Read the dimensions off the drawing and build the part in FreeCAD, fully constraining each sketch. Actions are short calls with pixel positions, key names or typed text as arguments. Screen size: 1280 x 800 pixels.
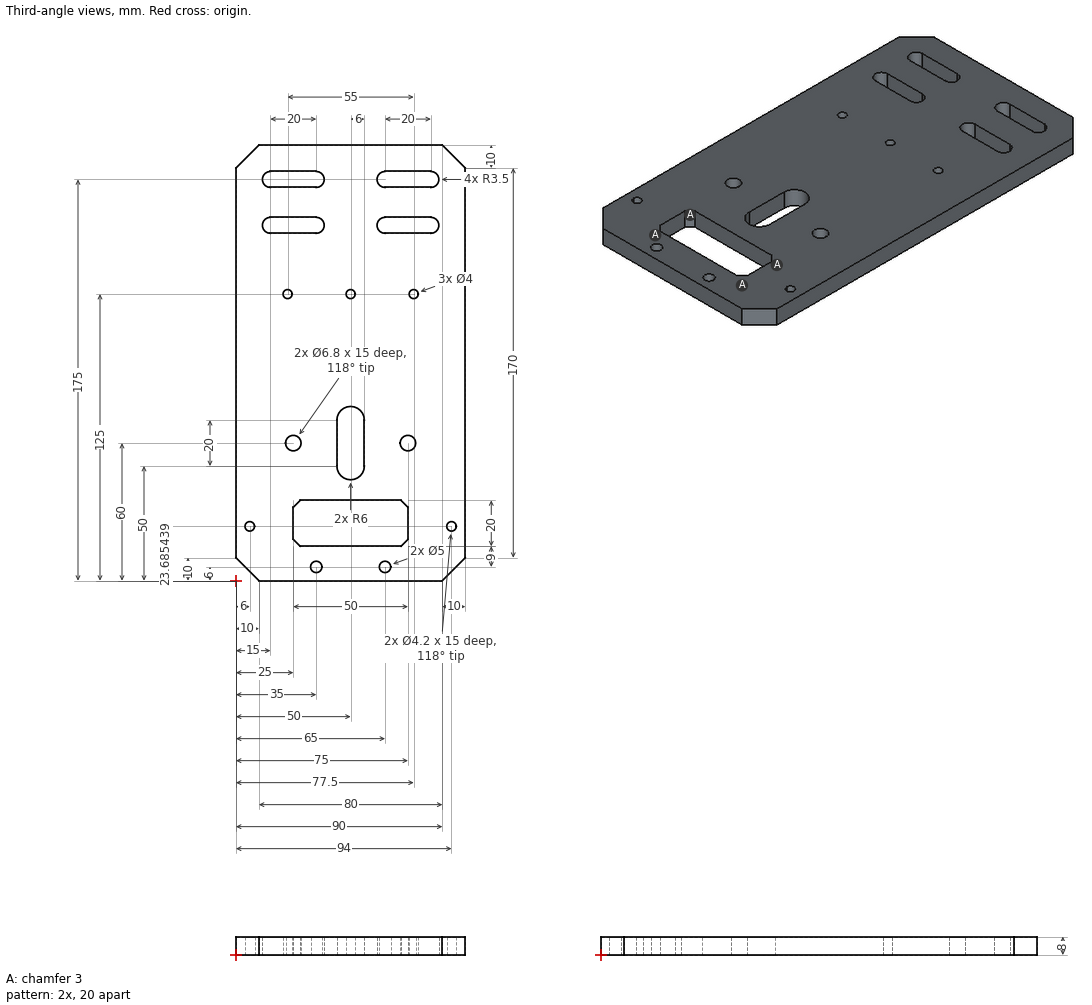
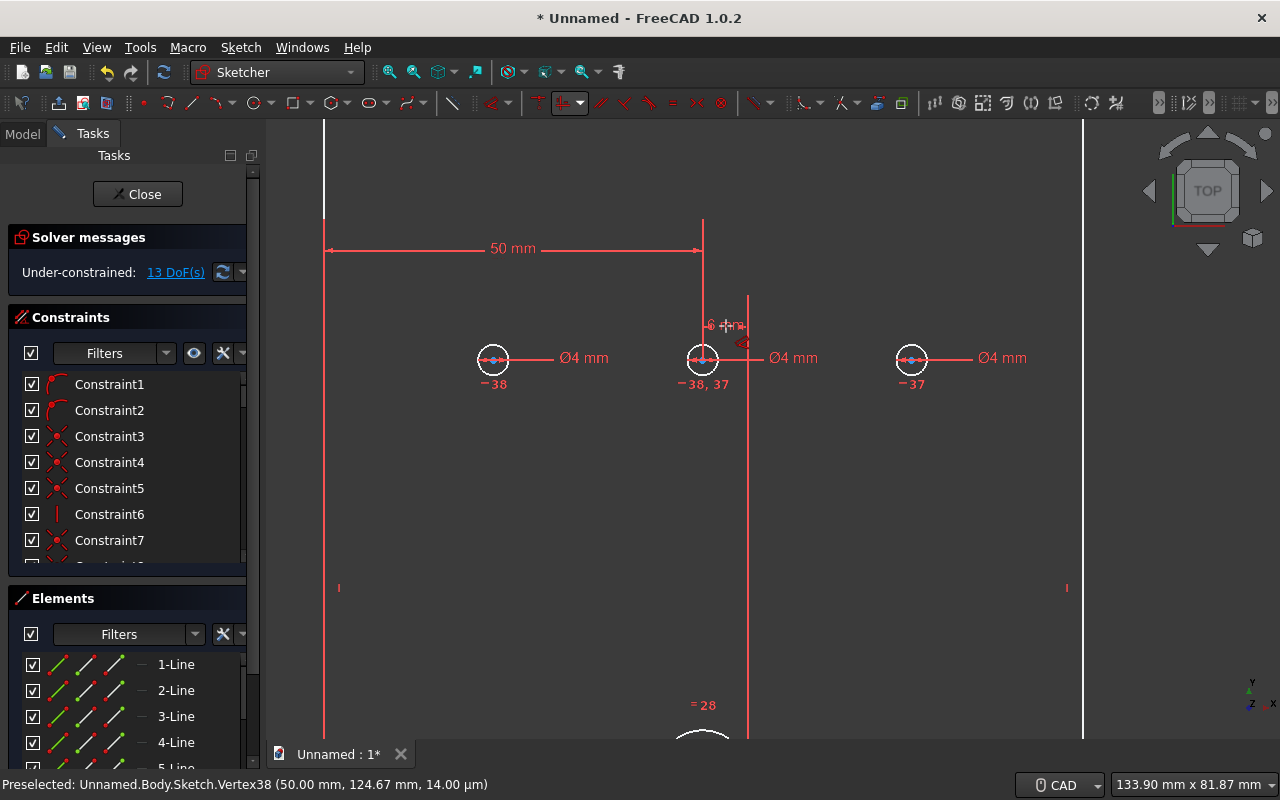
click(1083, 330)
click(1049, 429)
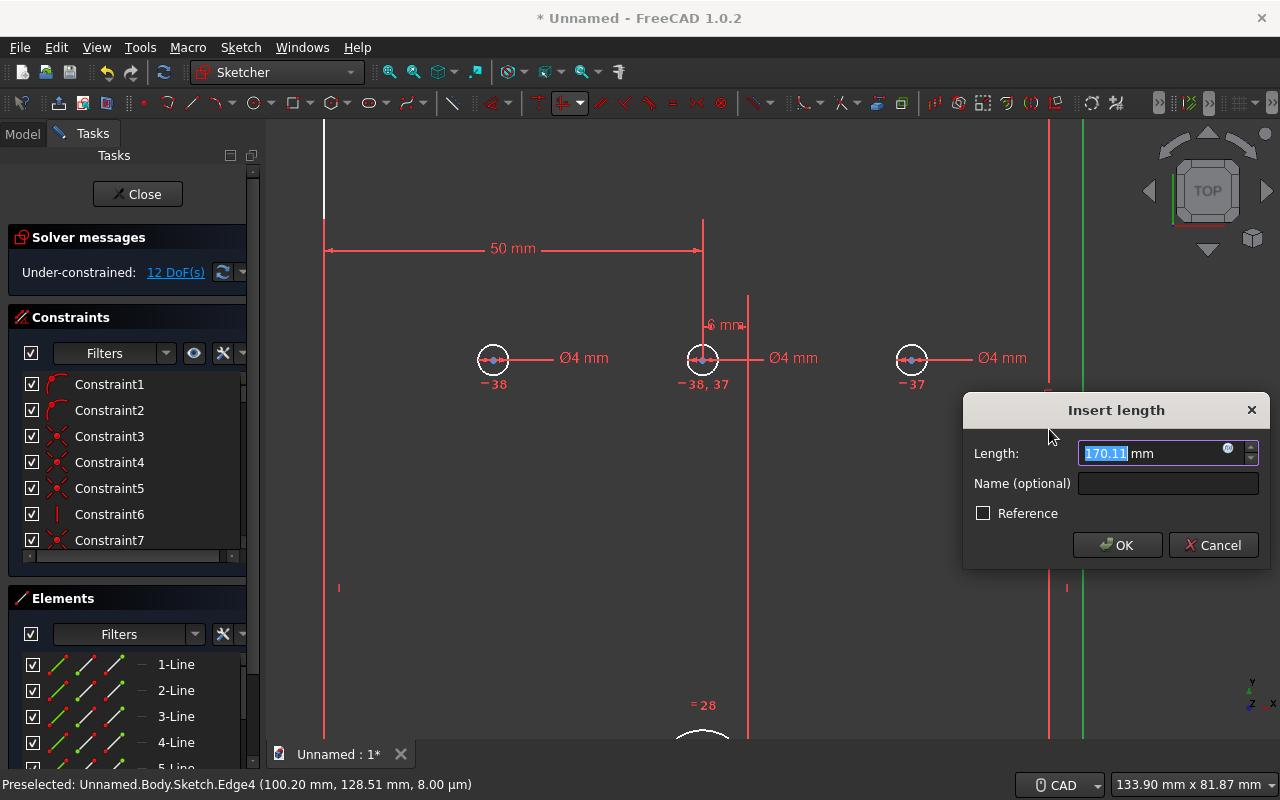
text(170)
key(Return)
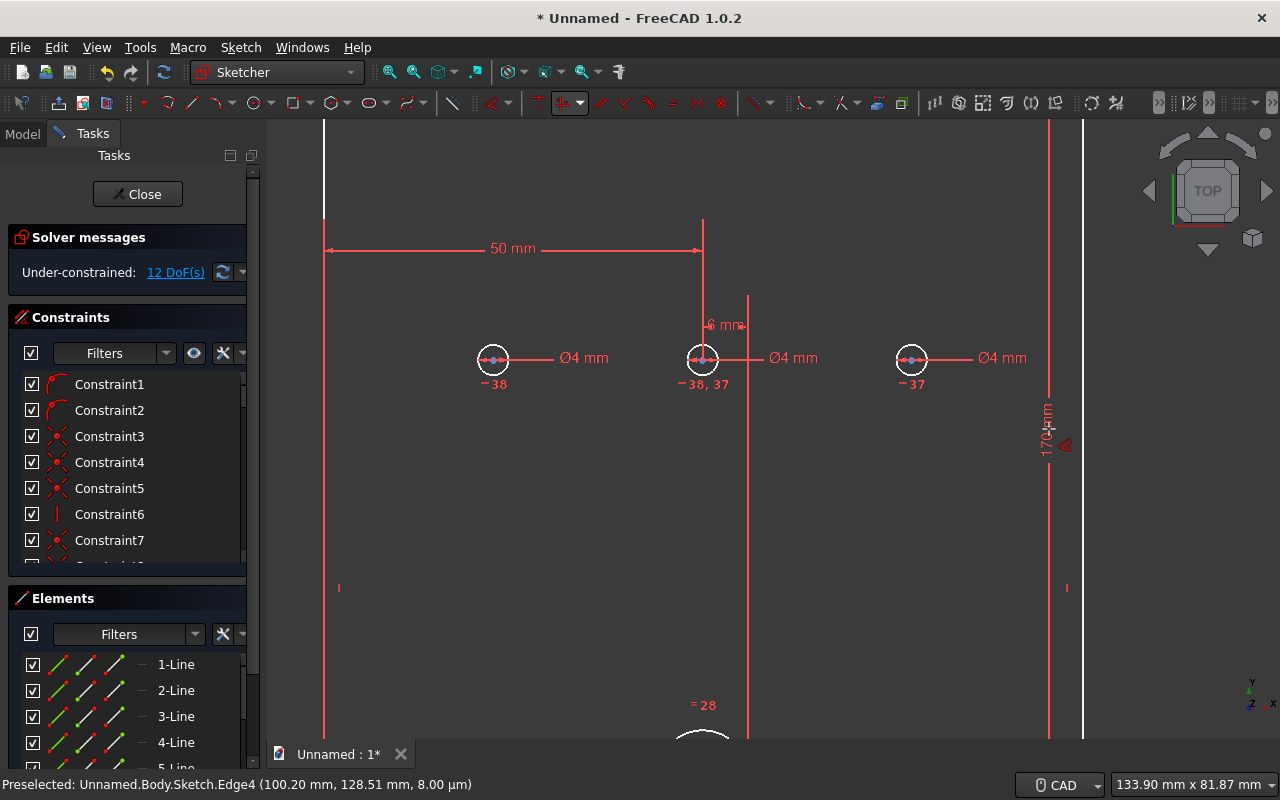
click(324, 330)
click(358, 429)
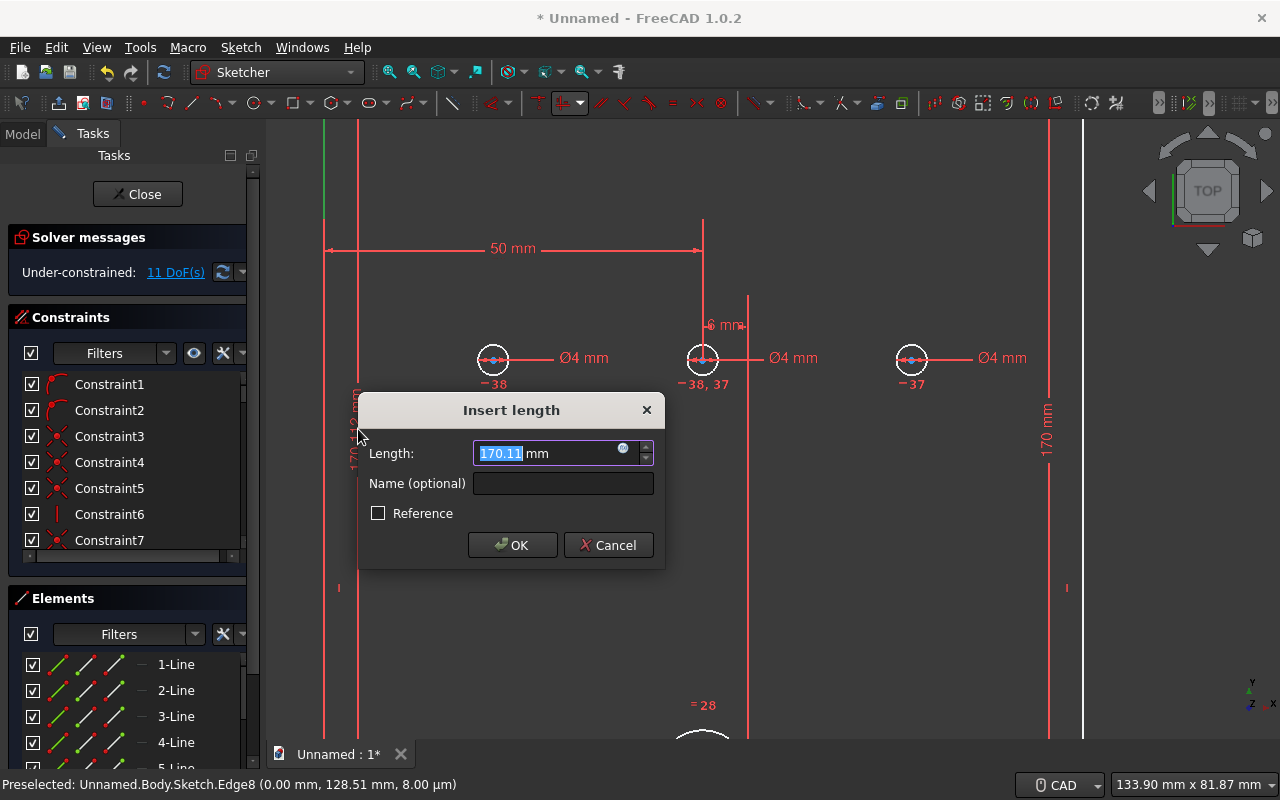
text(170)
key(Return)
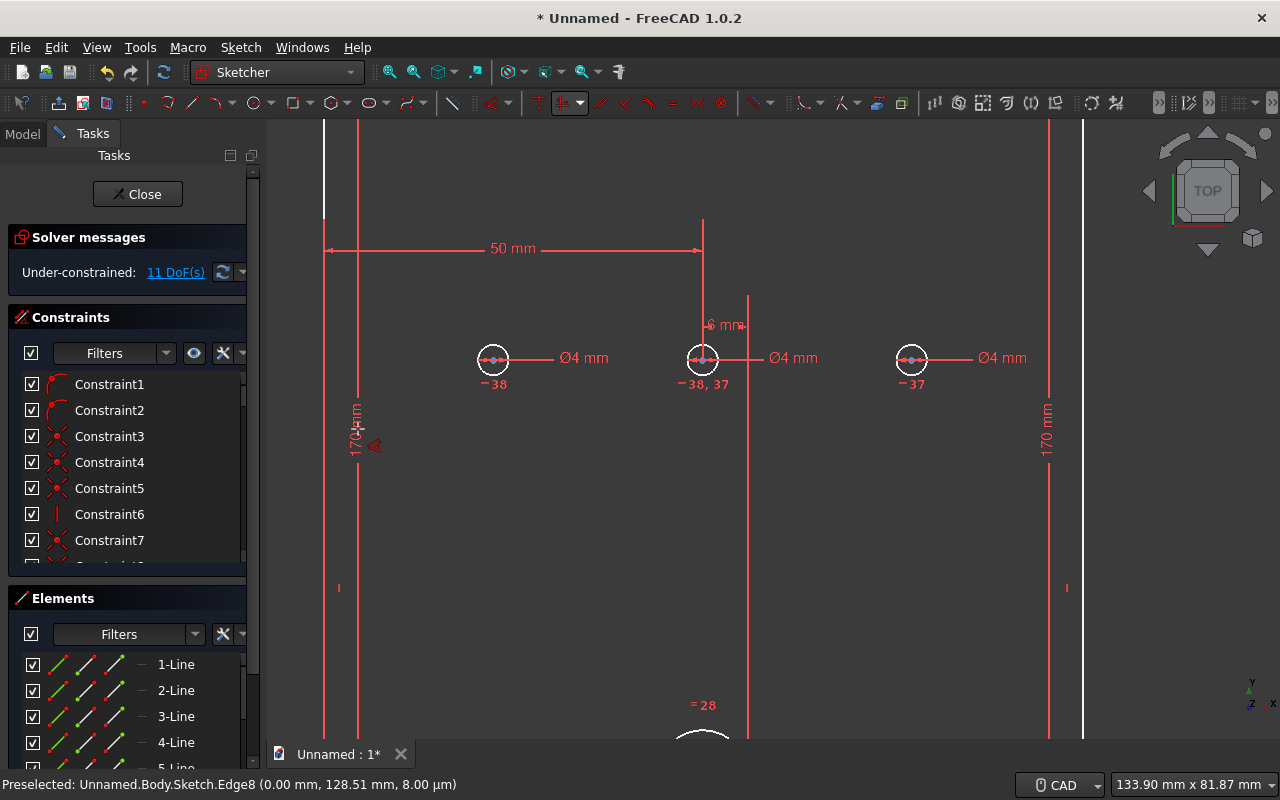
scroll(705, 362, down, 6)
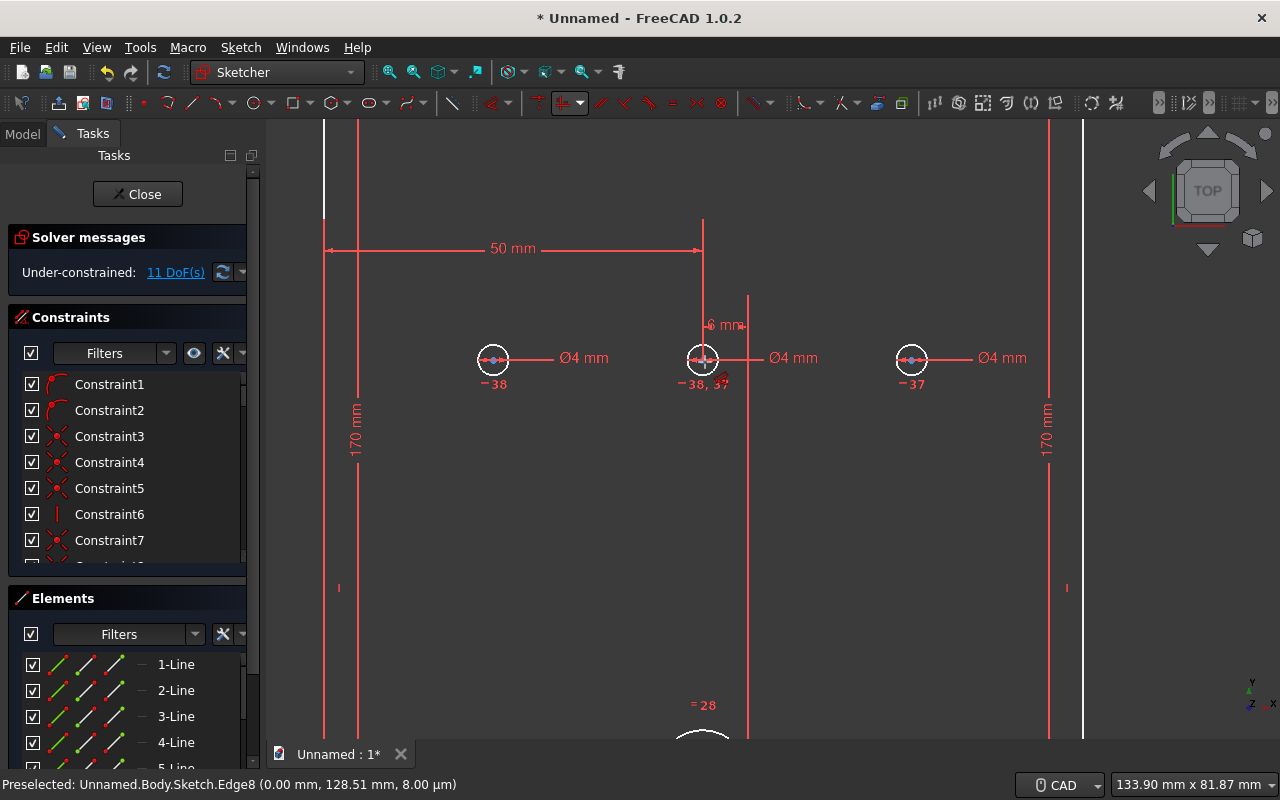
scroll(591, 624, up, 3)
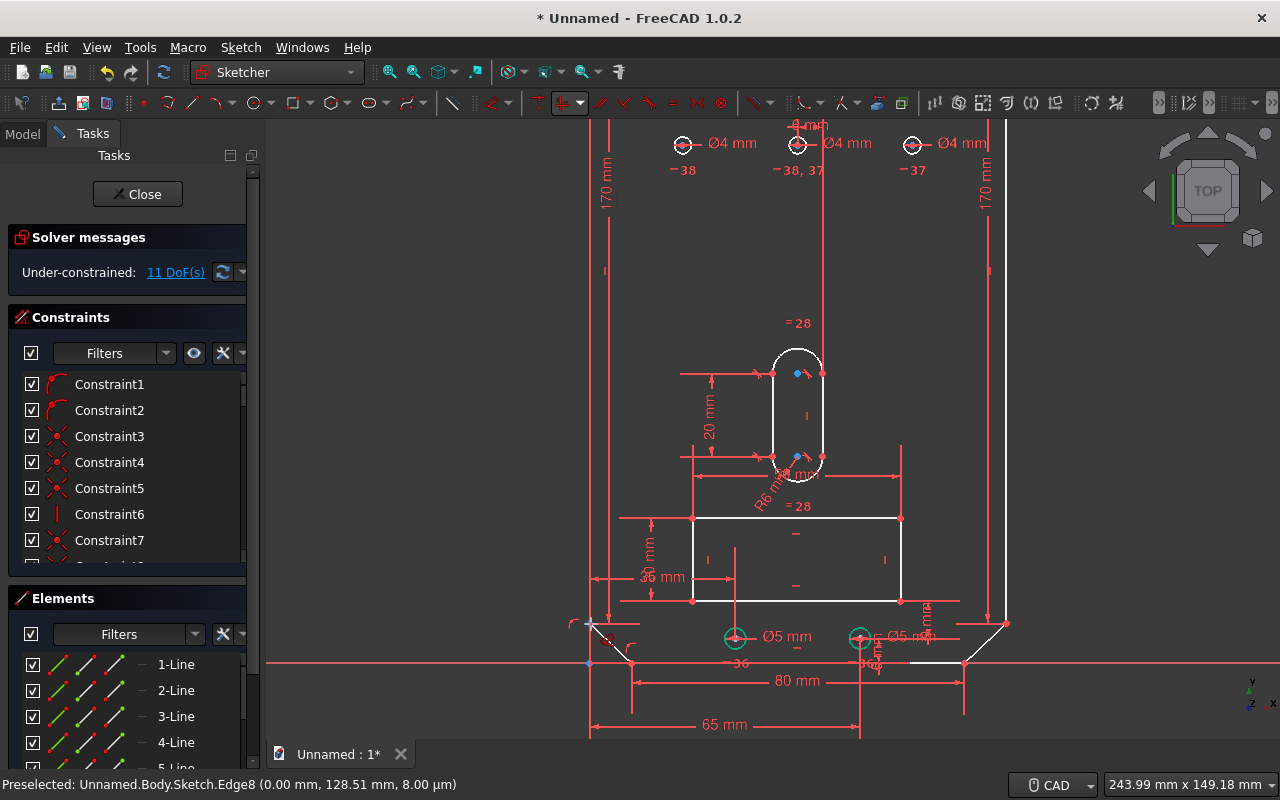
click(590, 624)
click(556, 644)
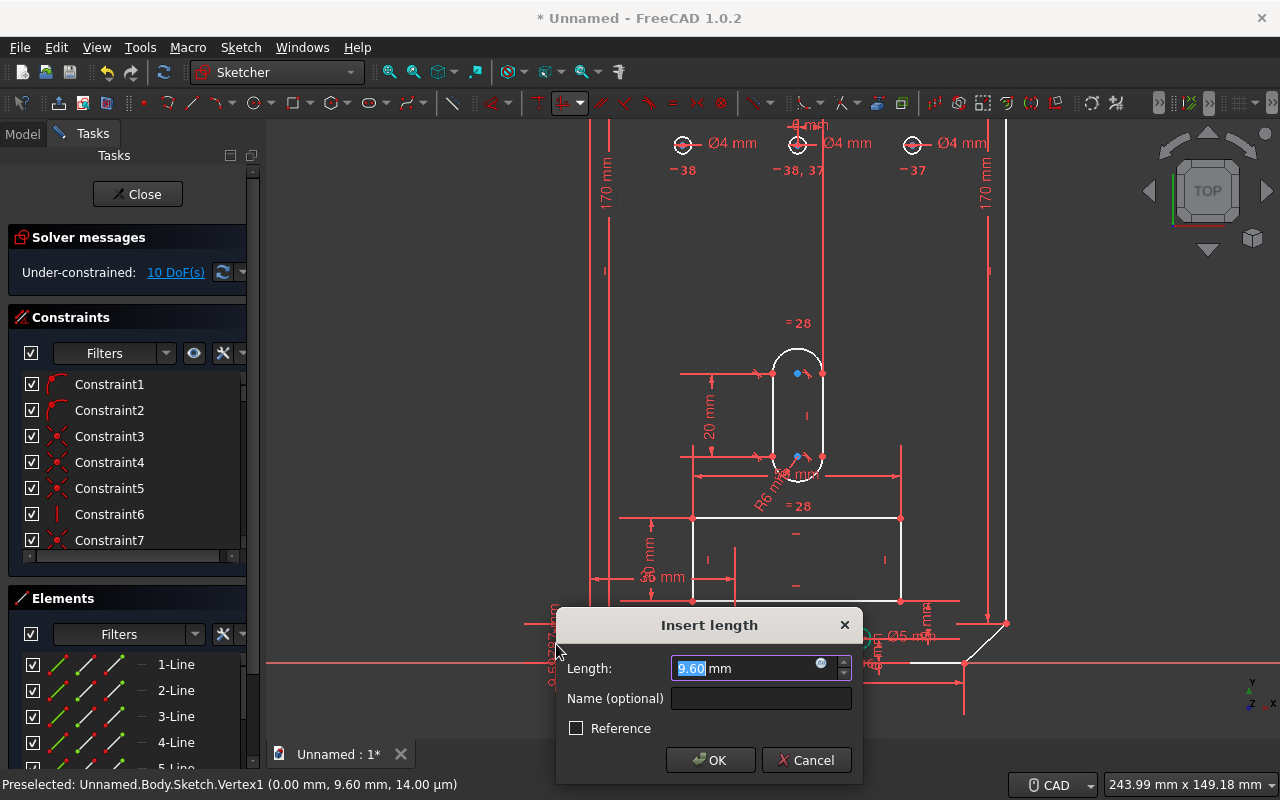
text(10)
key(Return)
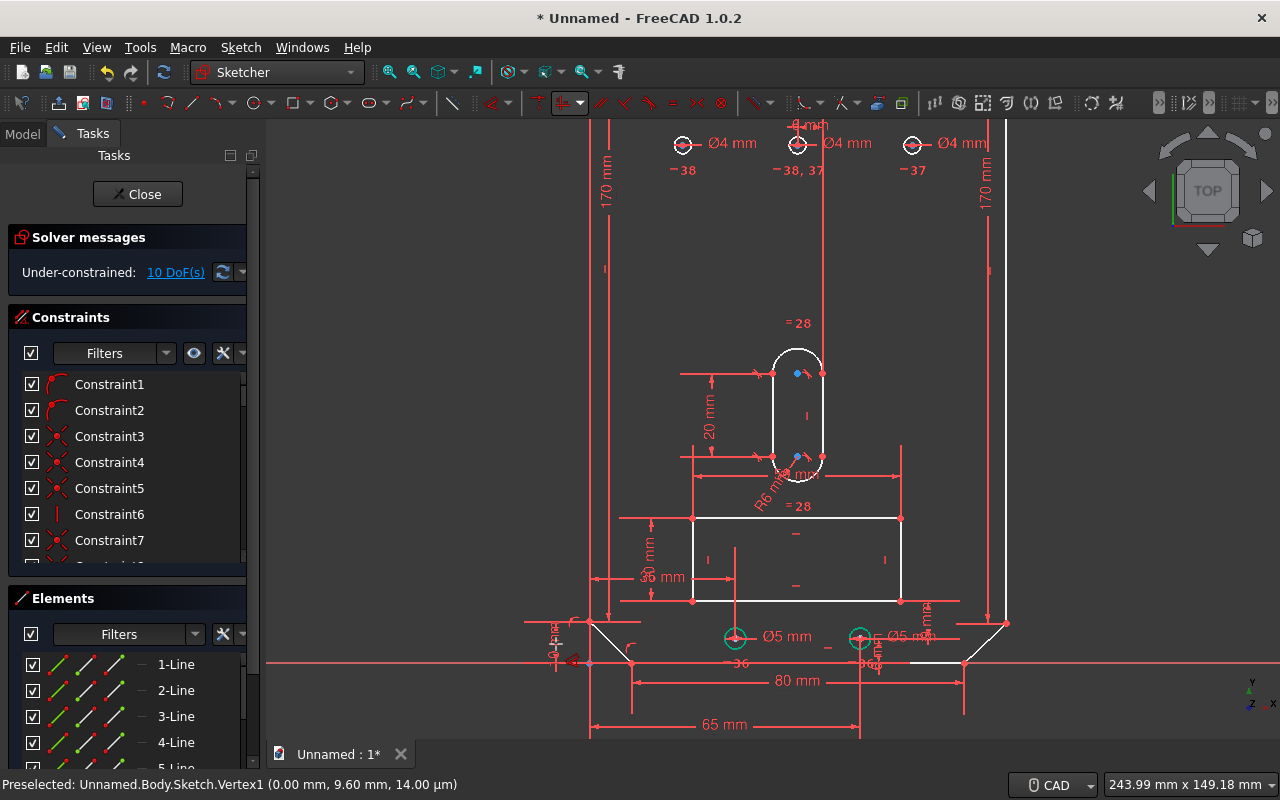
click(632, 663)
click(611, 697)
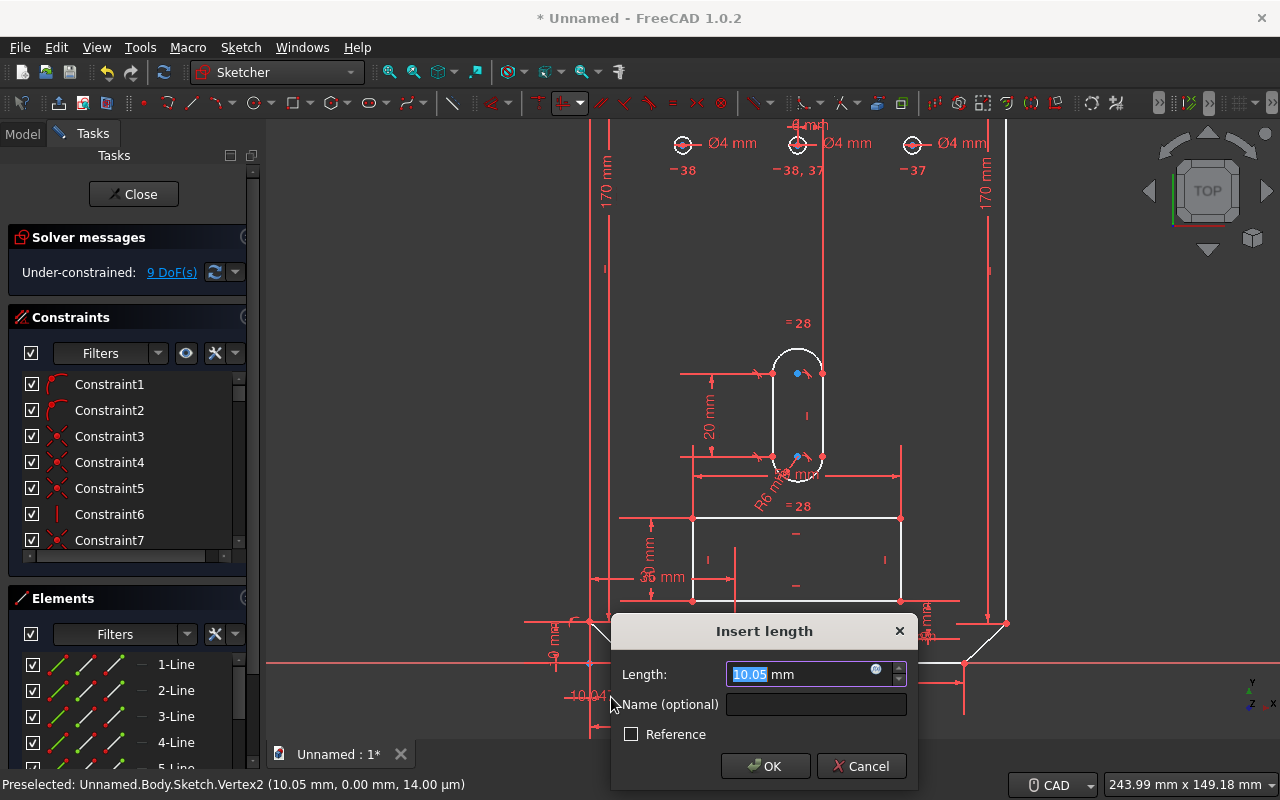
text(10)
key(Return)